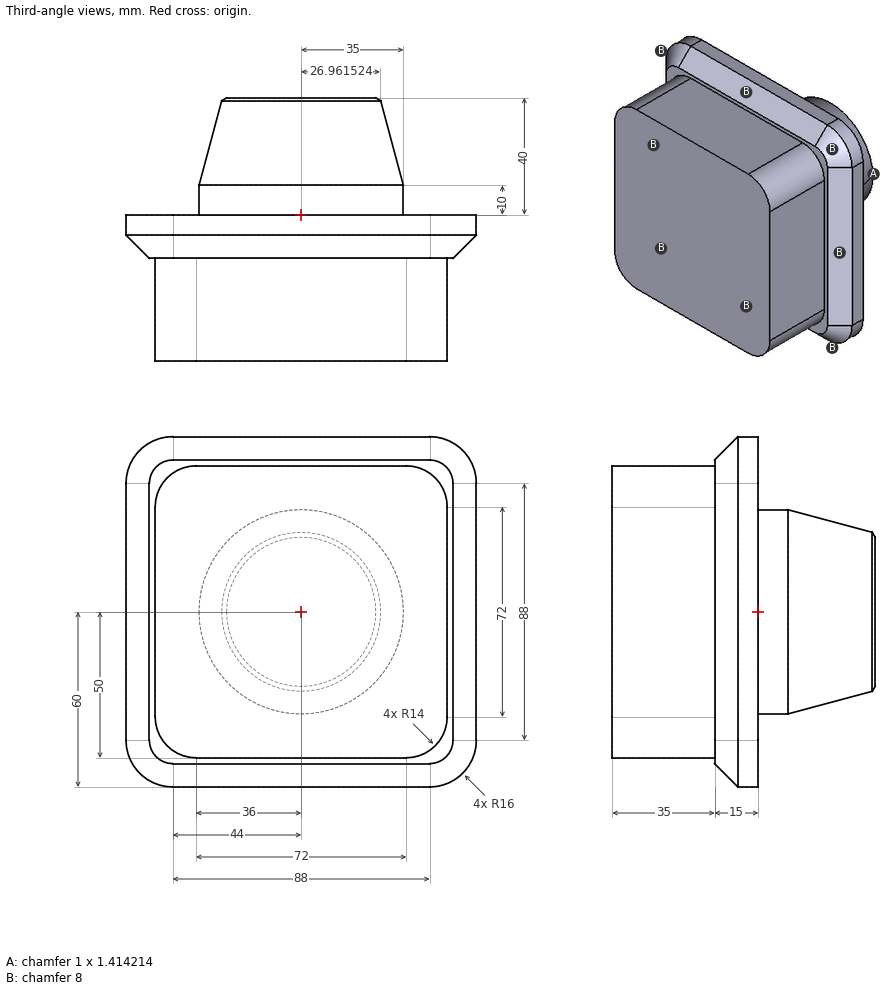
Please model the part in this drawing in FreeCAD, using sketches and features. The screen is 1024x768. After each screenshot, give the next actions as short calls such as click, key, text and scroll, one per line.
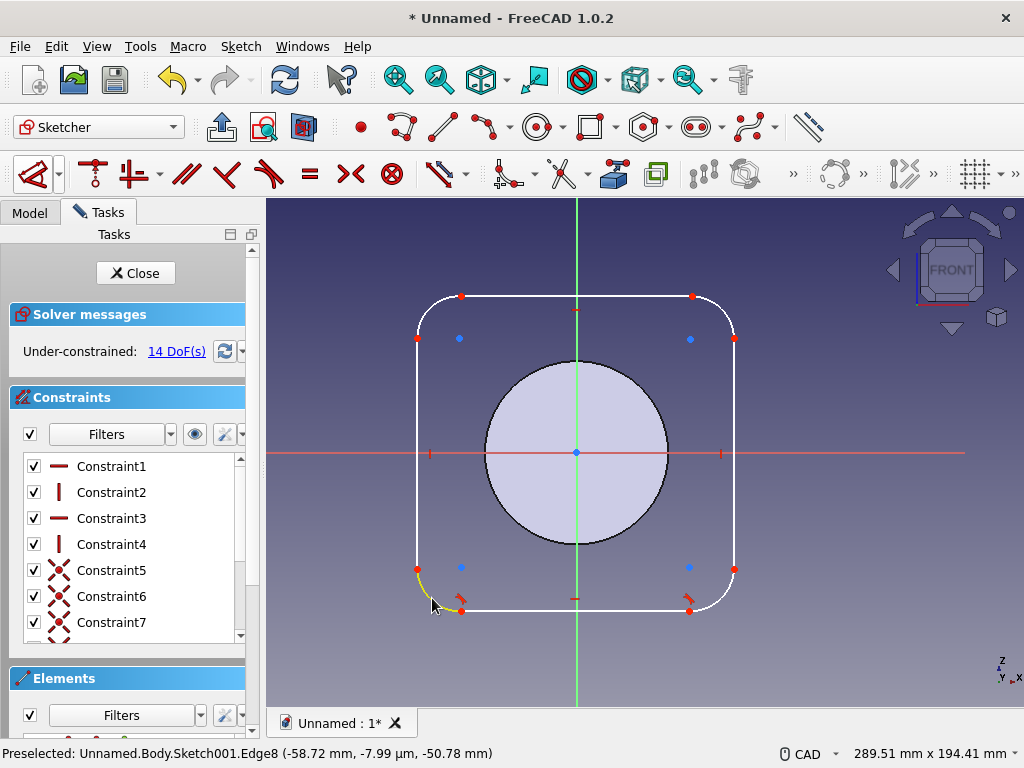
click(734, 500)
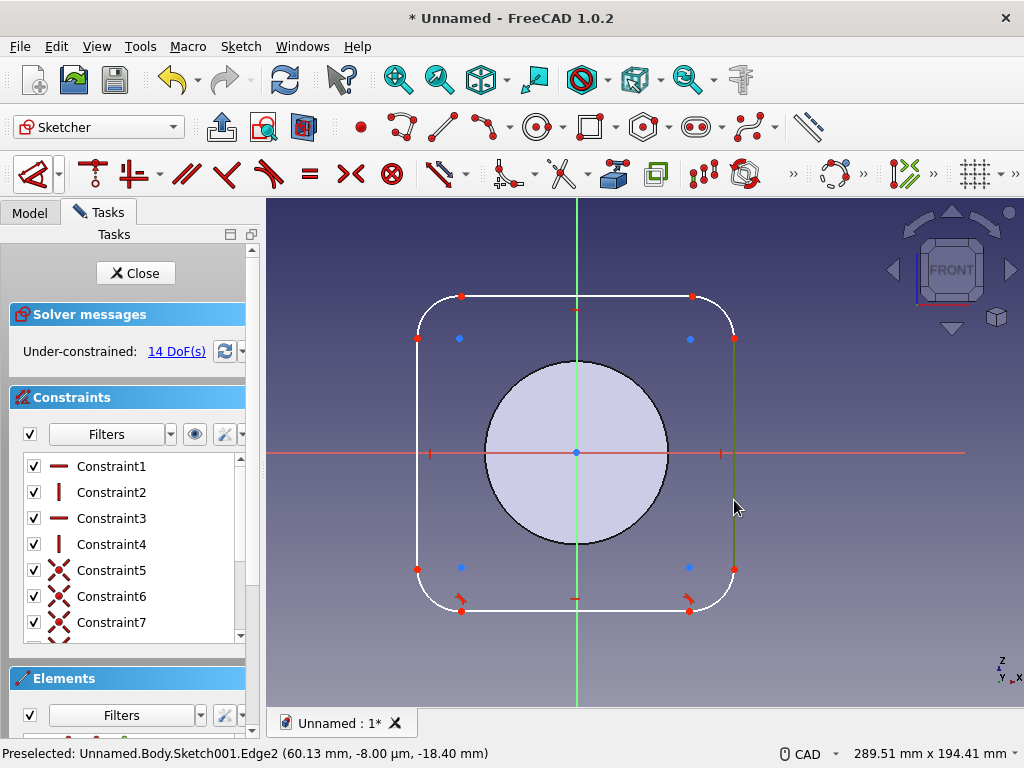
click(709, 607)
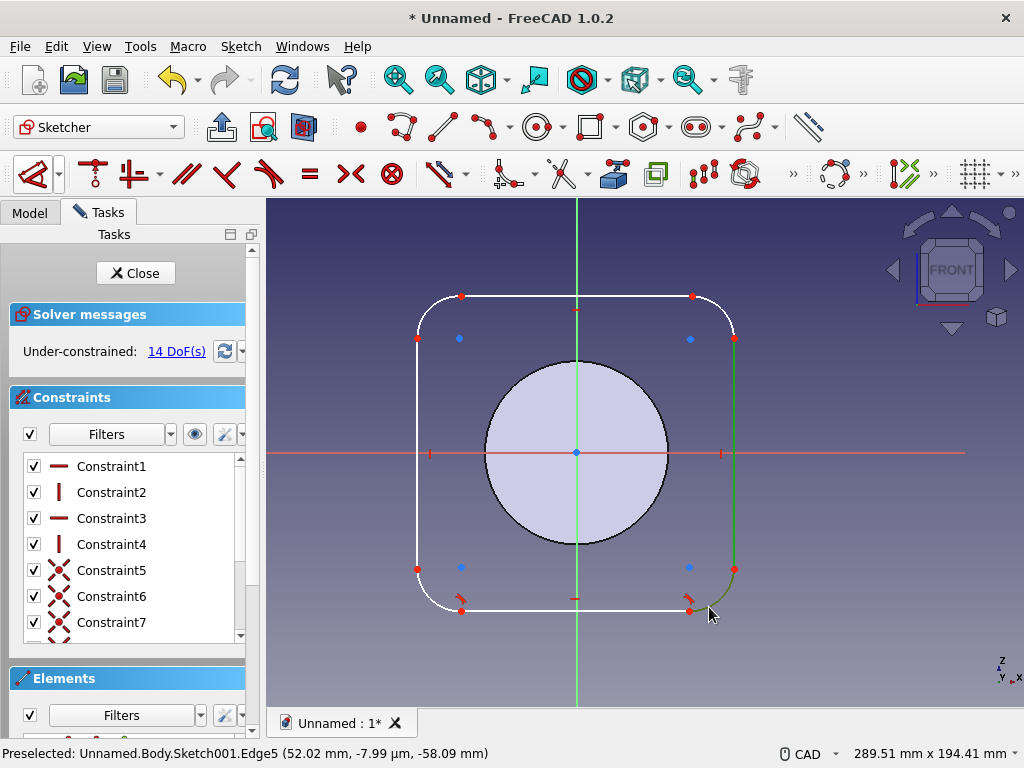
key(t)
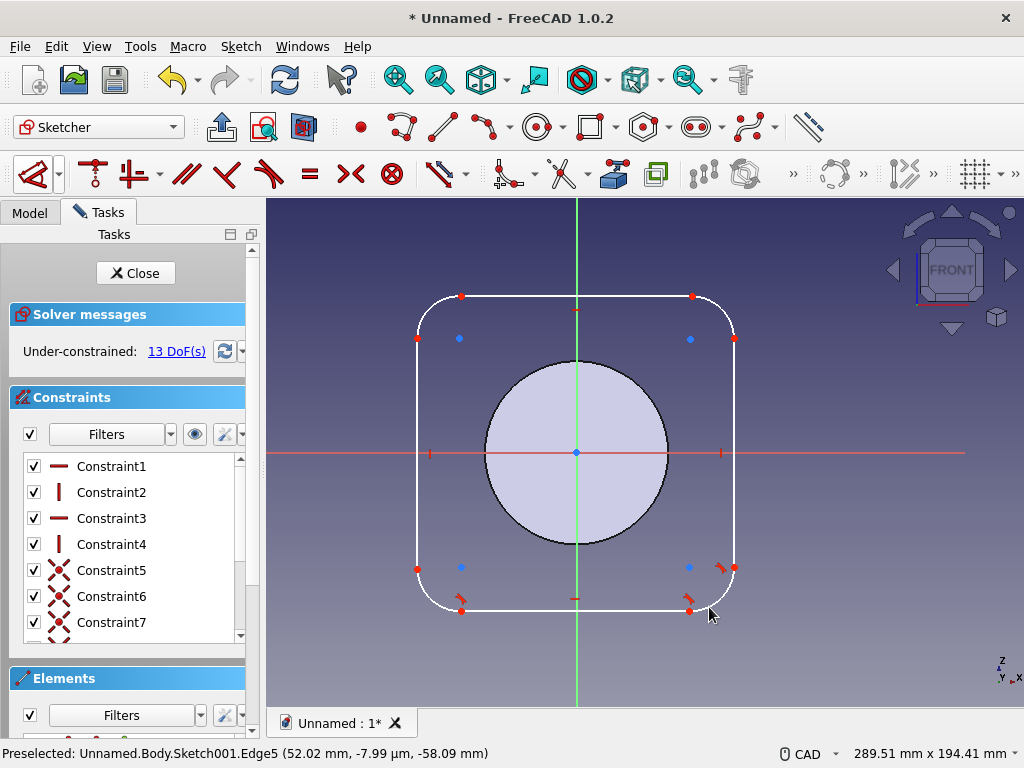
click(734, 498)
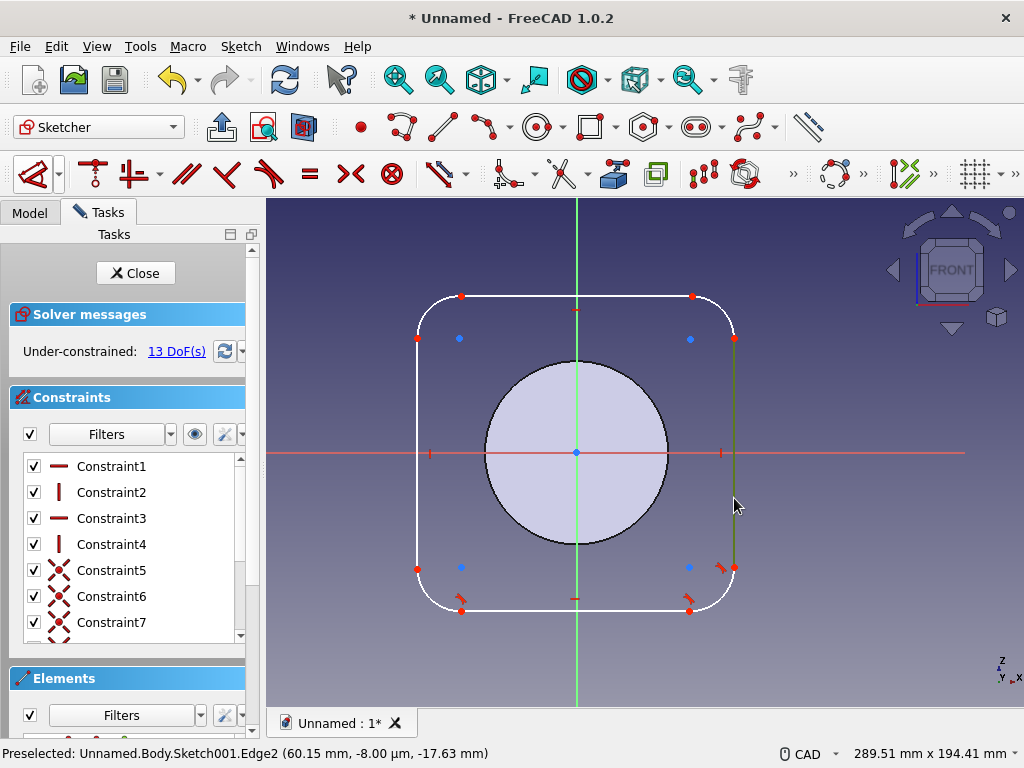
click(729, 319)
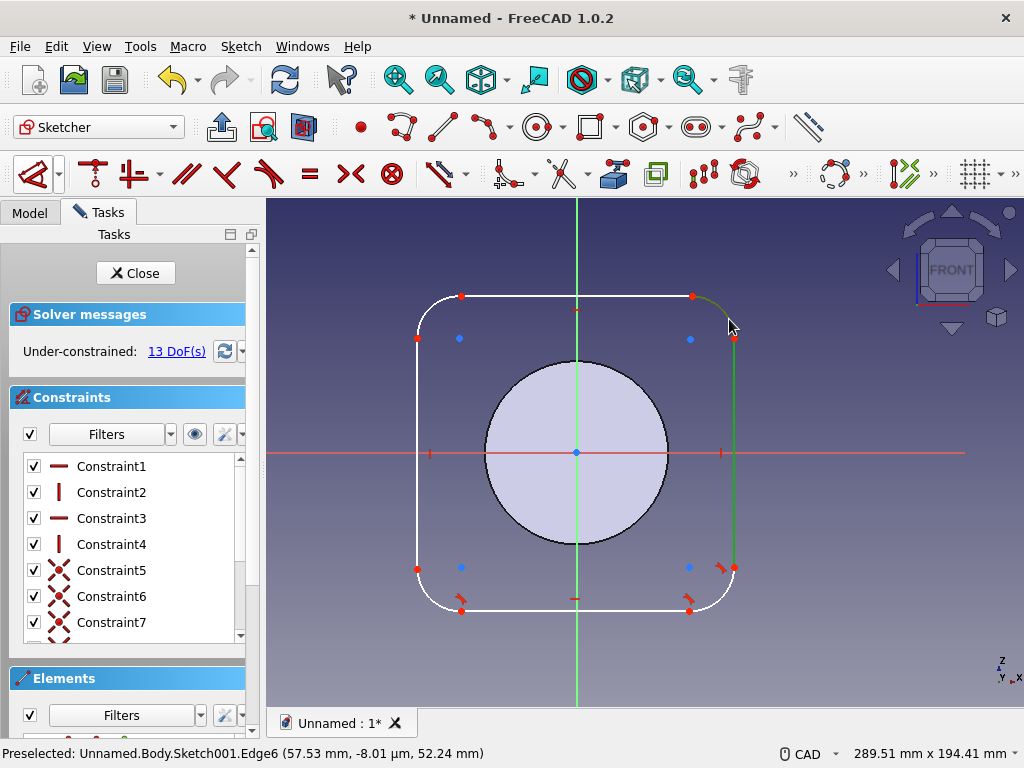
key(t)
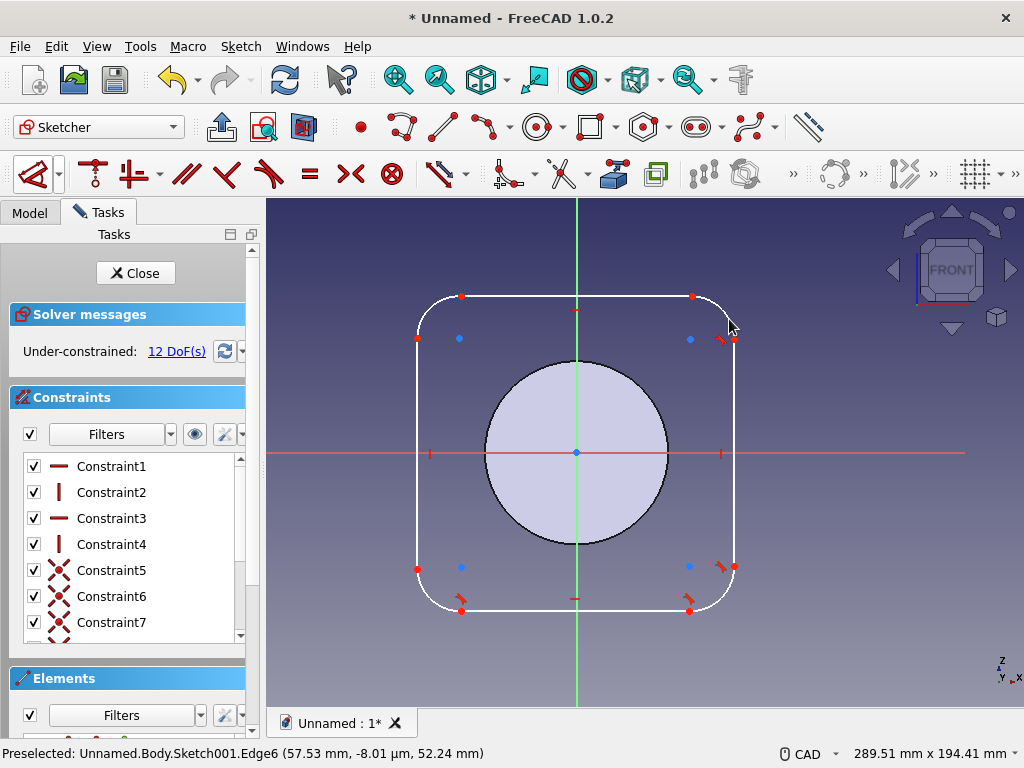
click(623, 296)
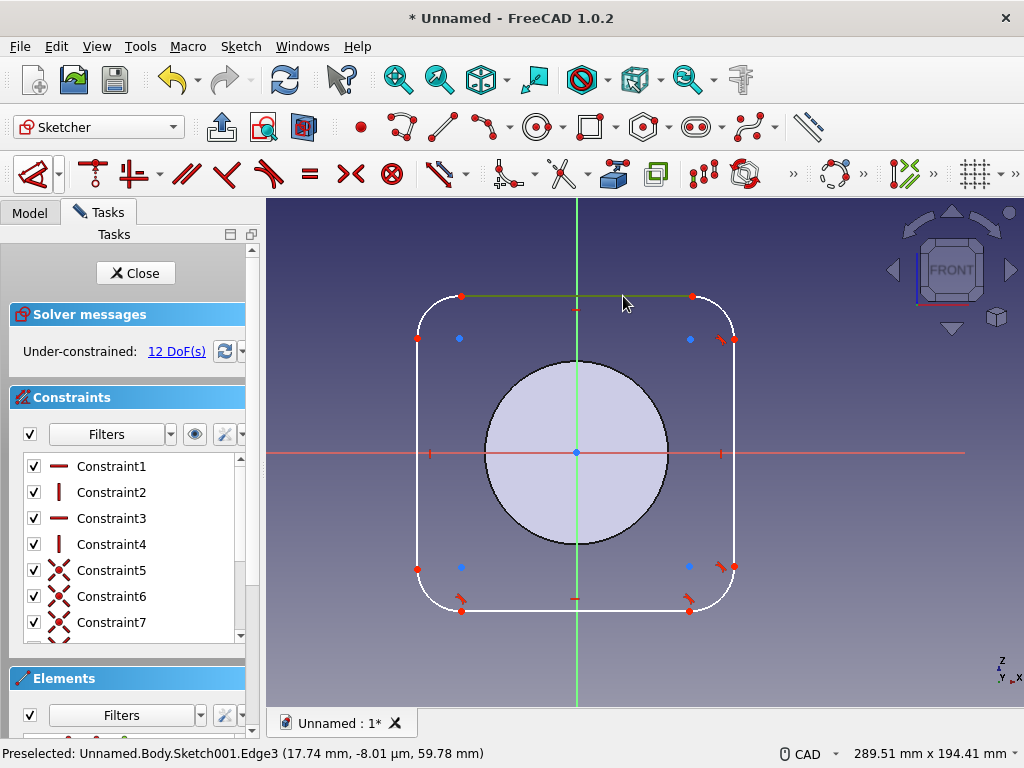
click(729, 320)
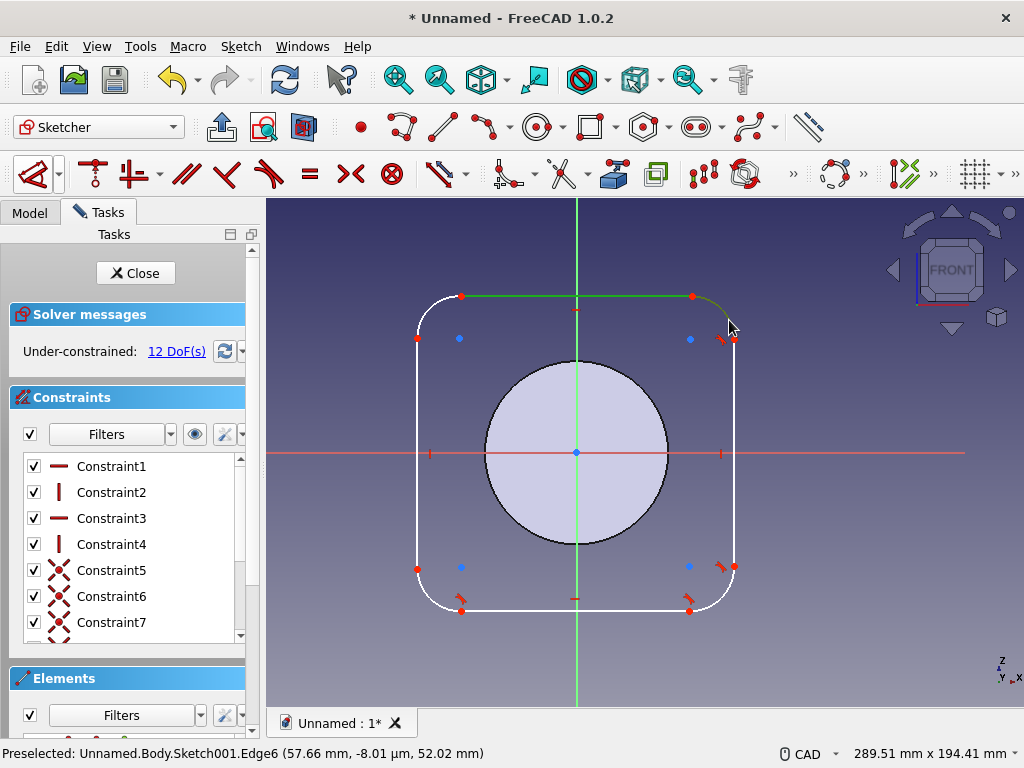
key(t)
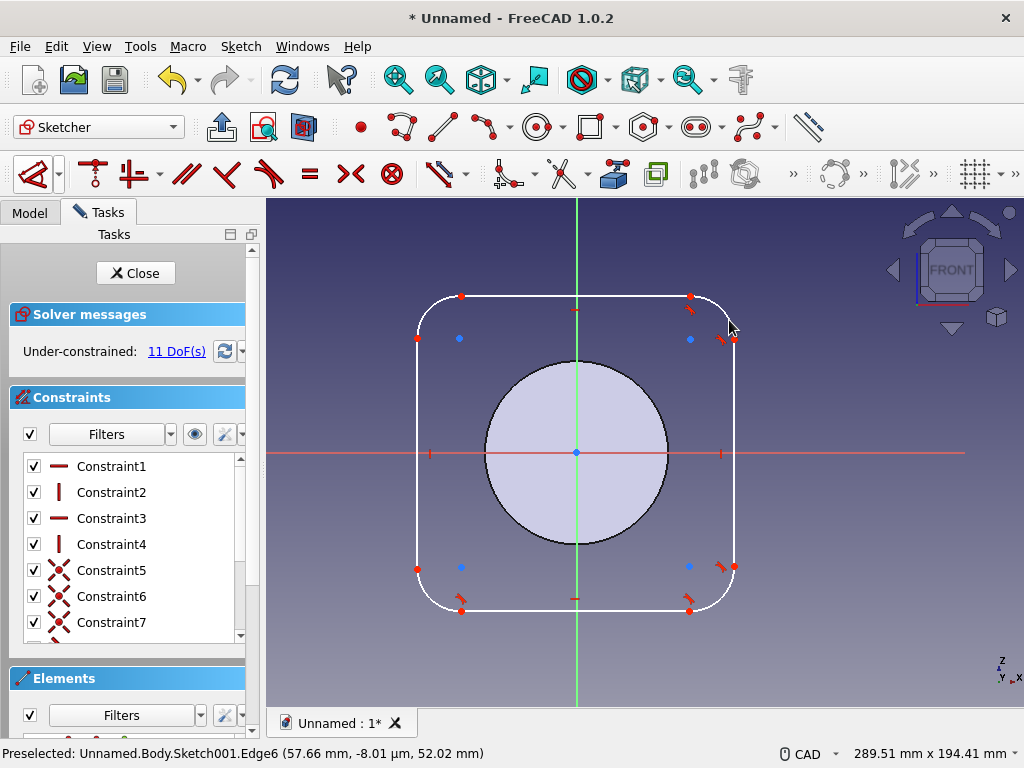
click(622, 296)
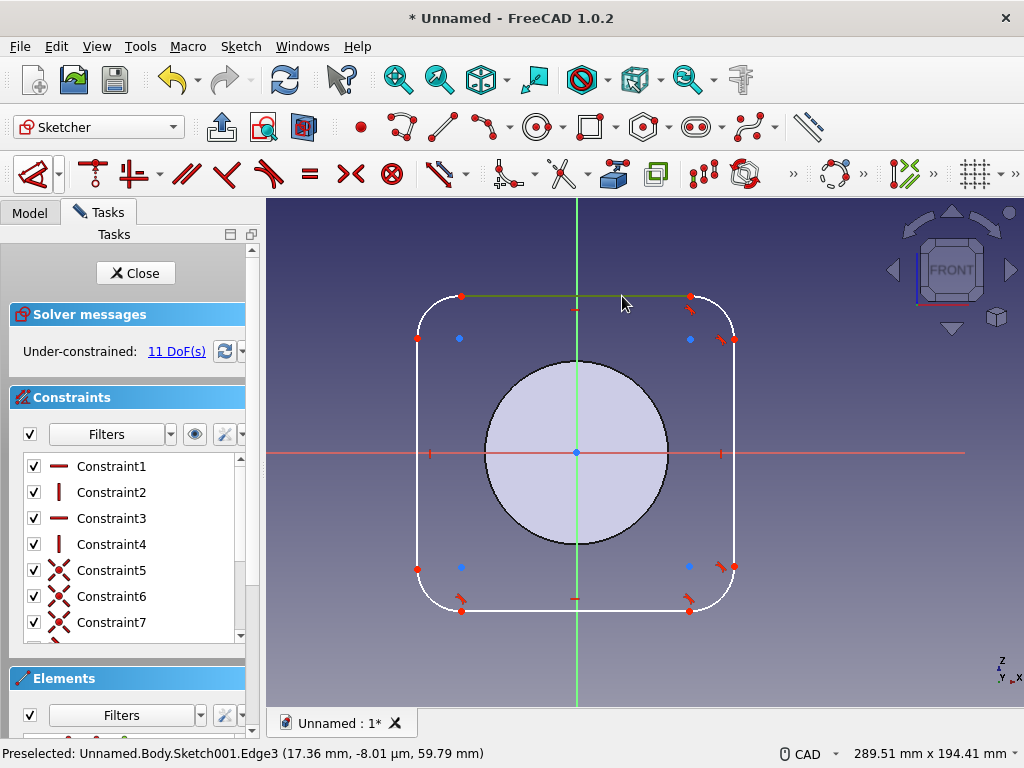
click(441, 300)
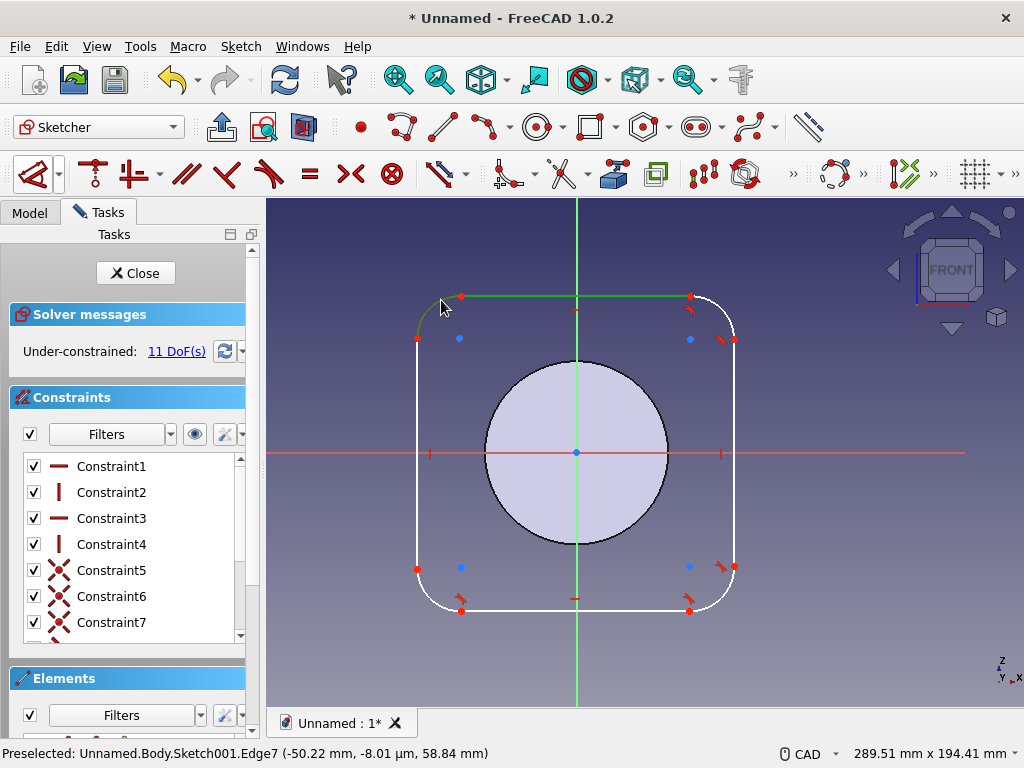
click(269, 174)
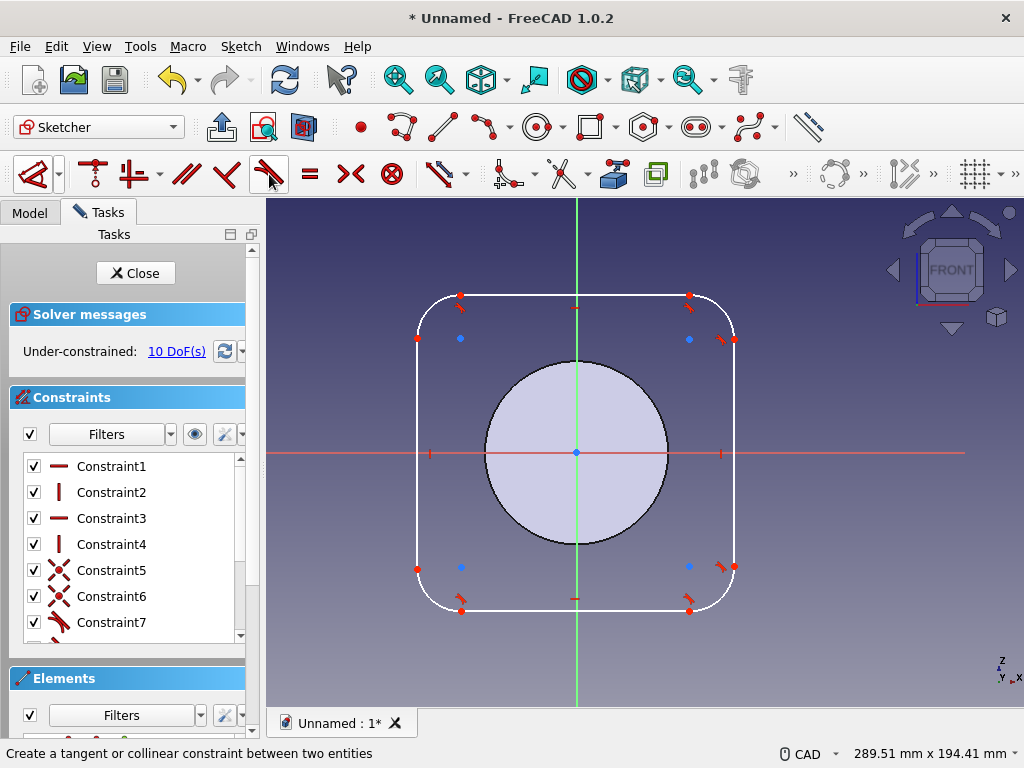
click(417, 408)